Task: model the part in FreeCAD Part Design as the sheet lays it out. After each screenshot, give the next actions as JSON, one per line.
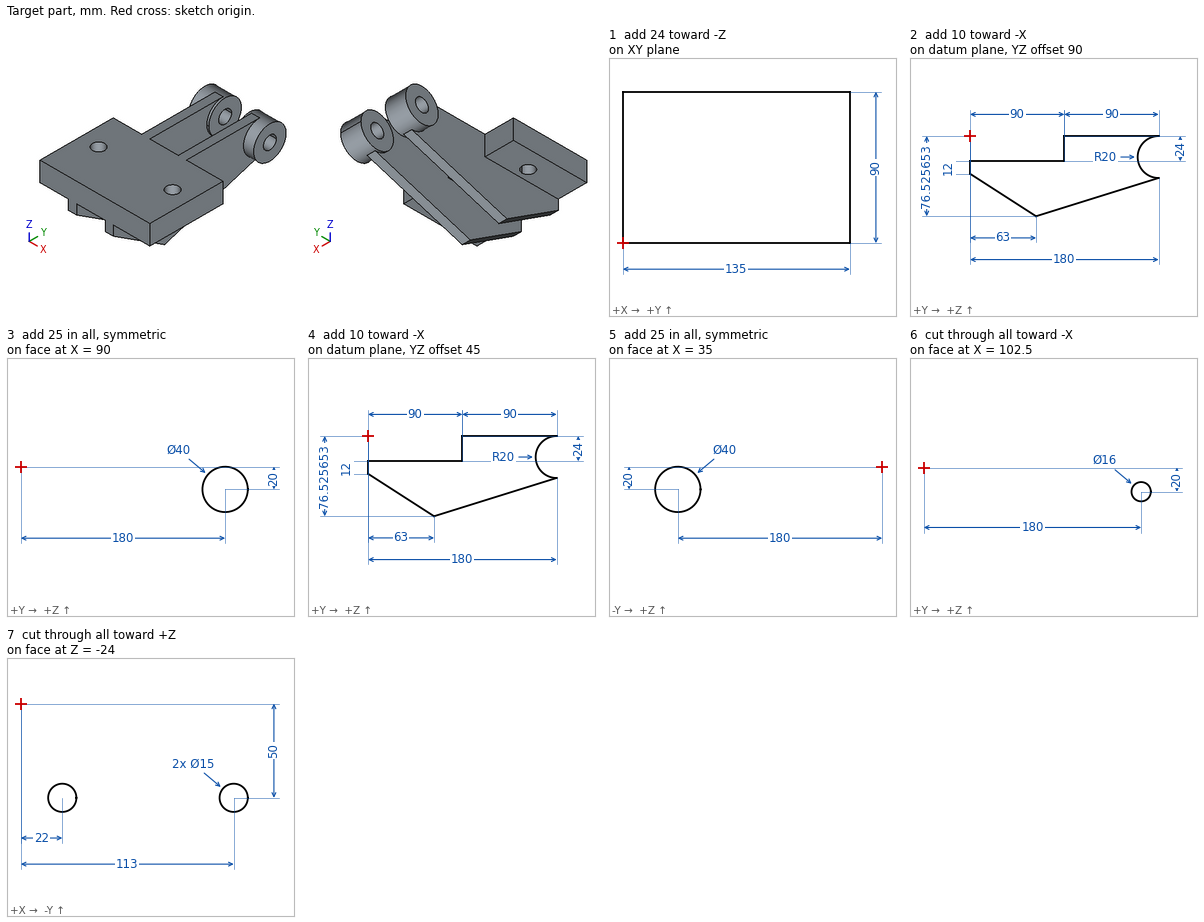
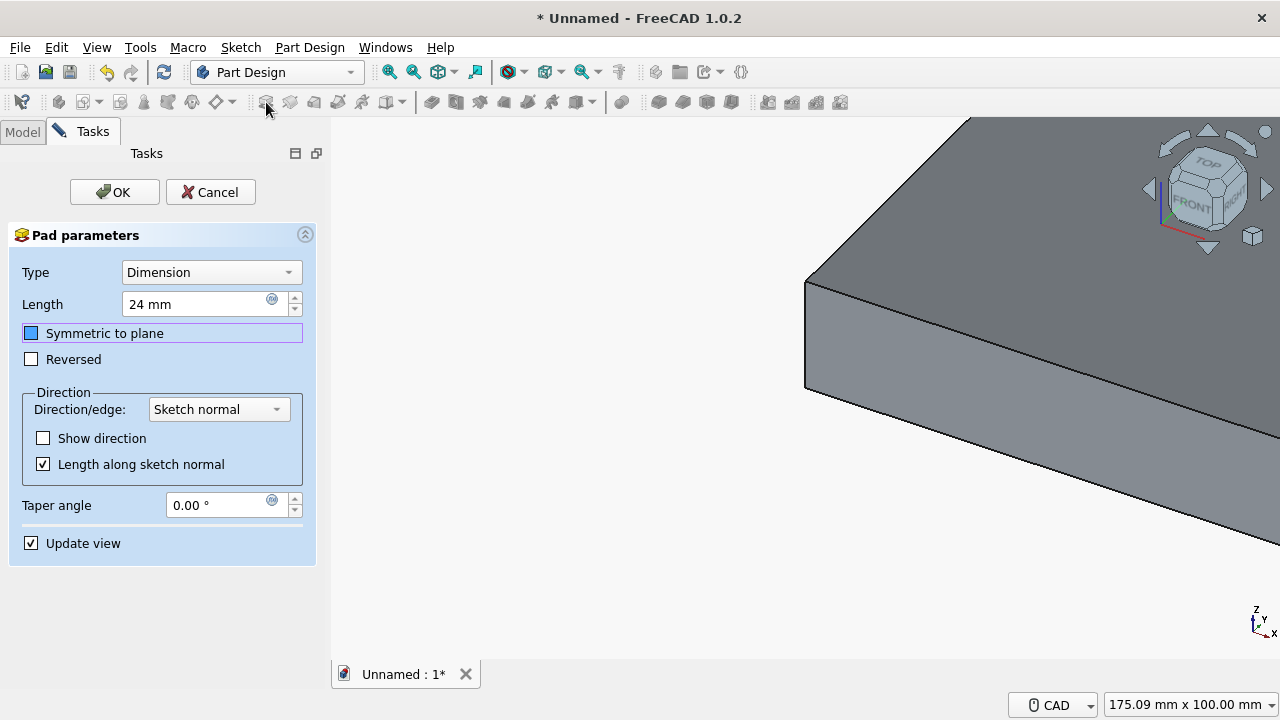
{"action": "left_click", "coordinate": [30, 359]}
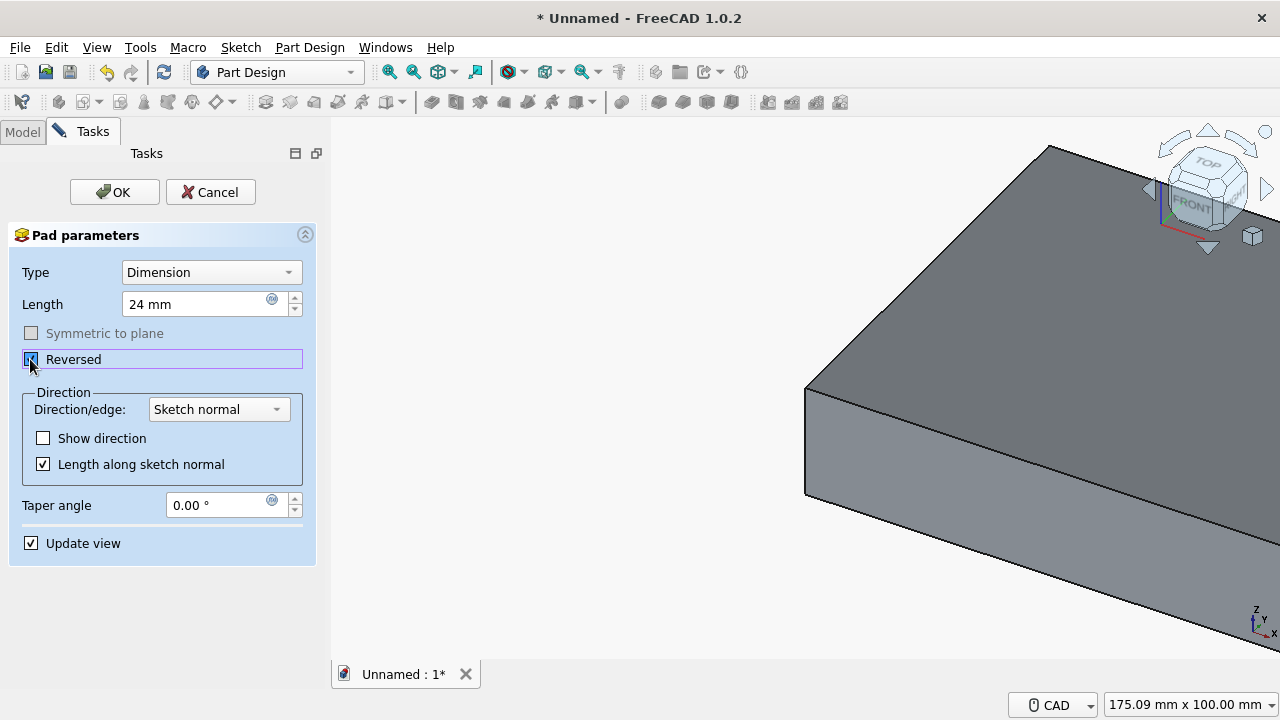
{"action": "left_click", "coordinate": [115, 192]}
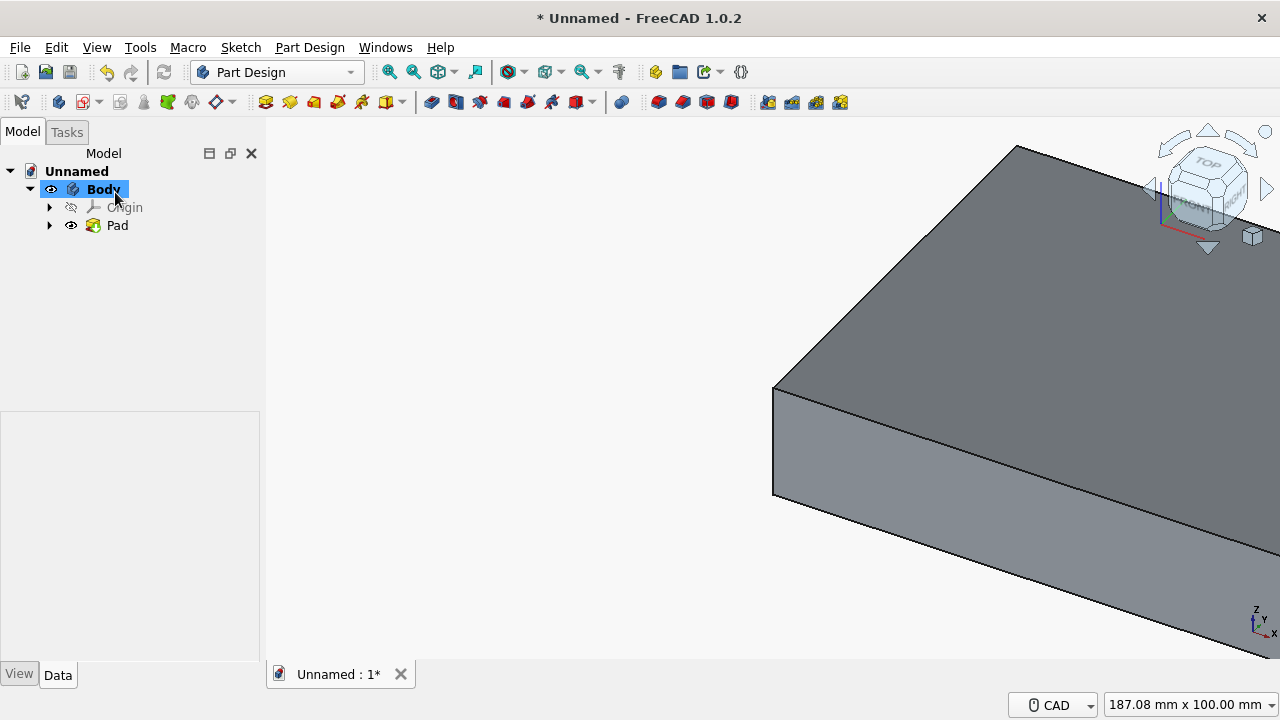
{"action": "left_click", "coordinate": [390, 72]}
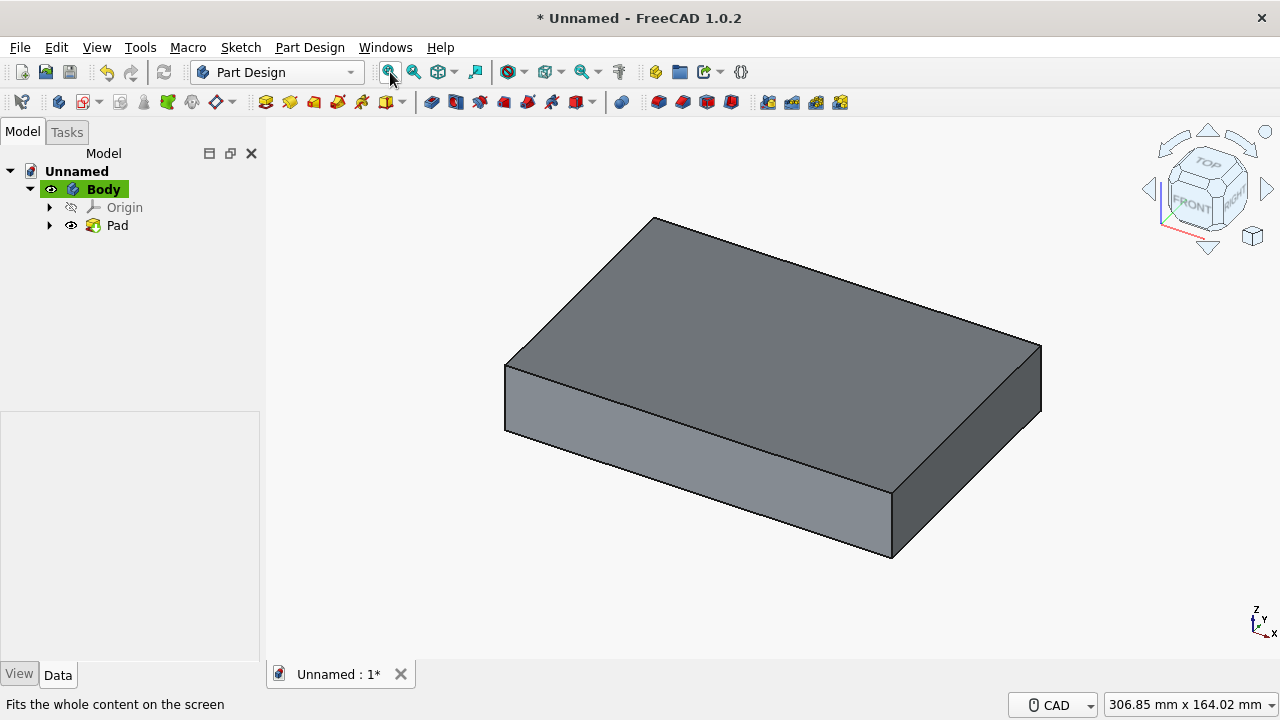
{"action": "left_click", "coordinate": [50, 207]}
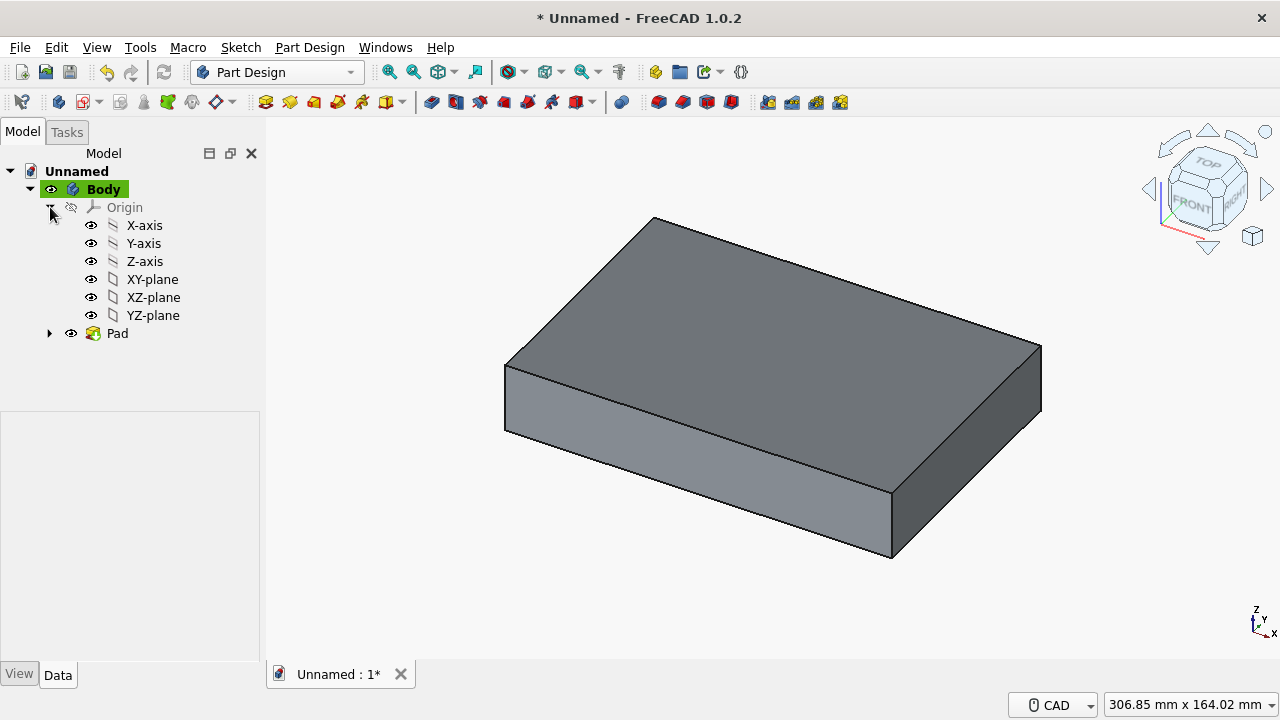
{"action": "left_click", "coordinate": [136, 315]}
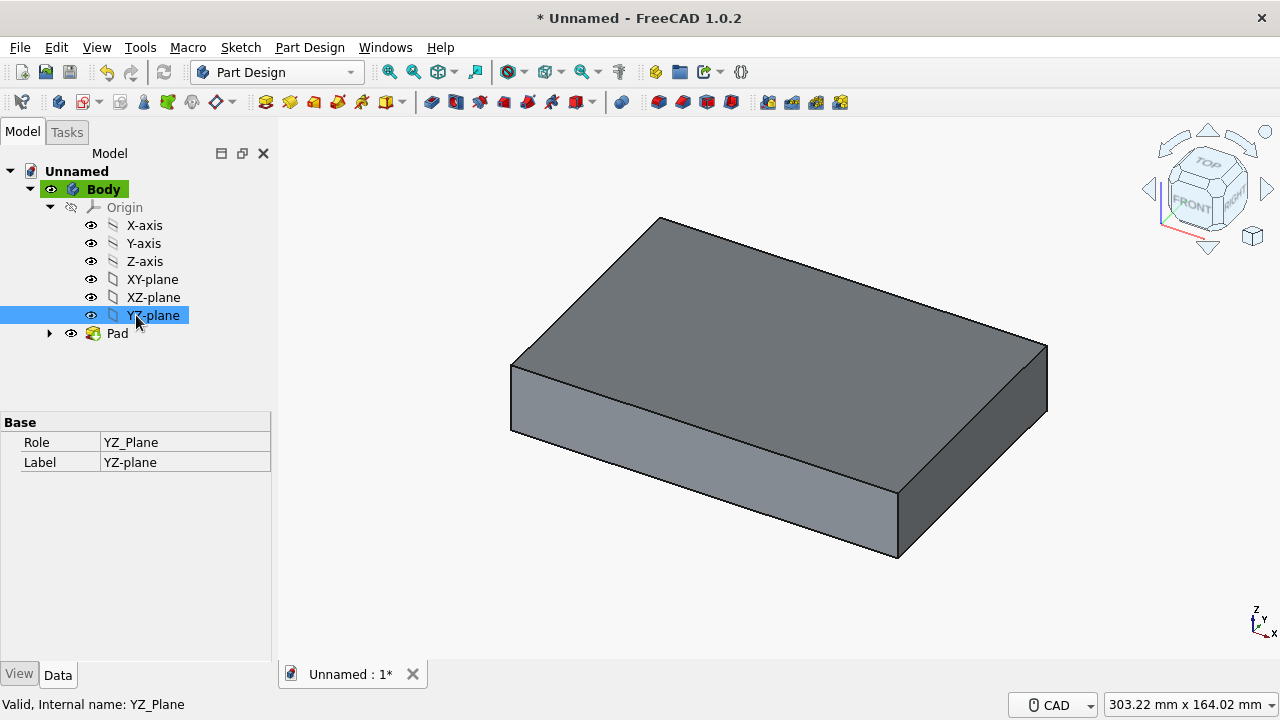
{"action": "left_click", "coordinate": [216, 102]}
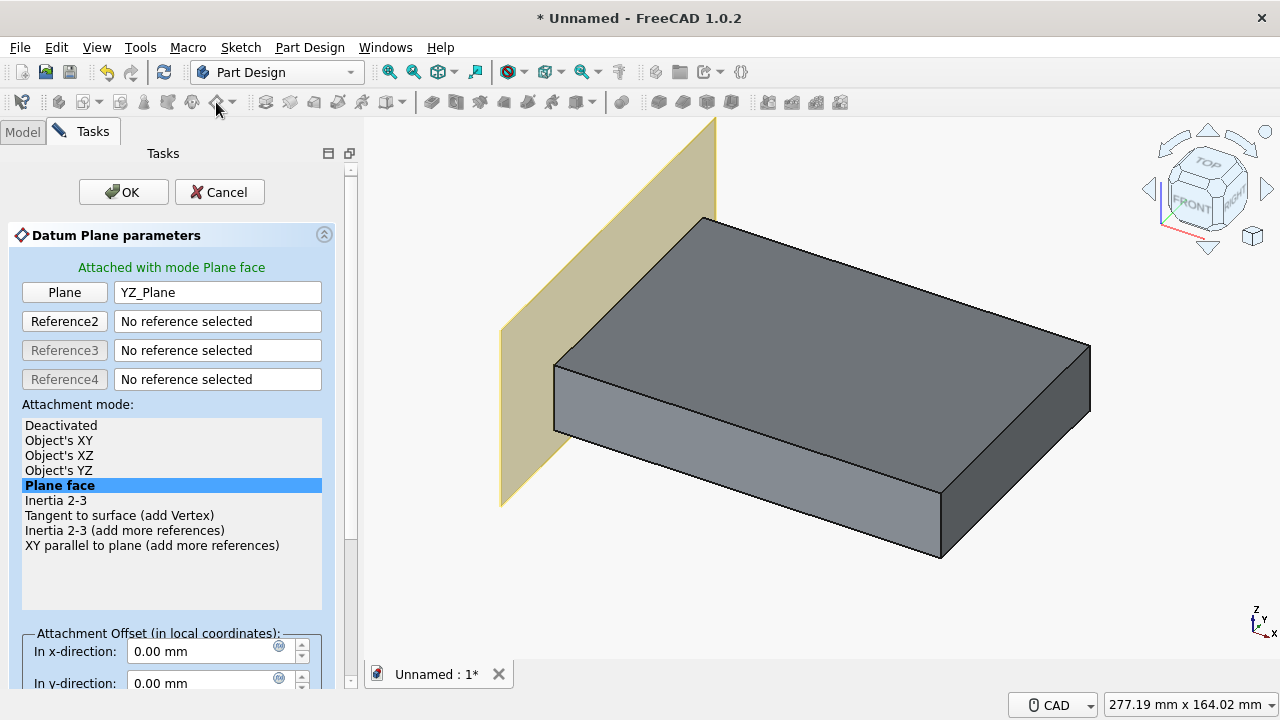
{"action": "scroll", "coordinate": [351, 426], "scroll_direction": "down", "scroll_amount": 2}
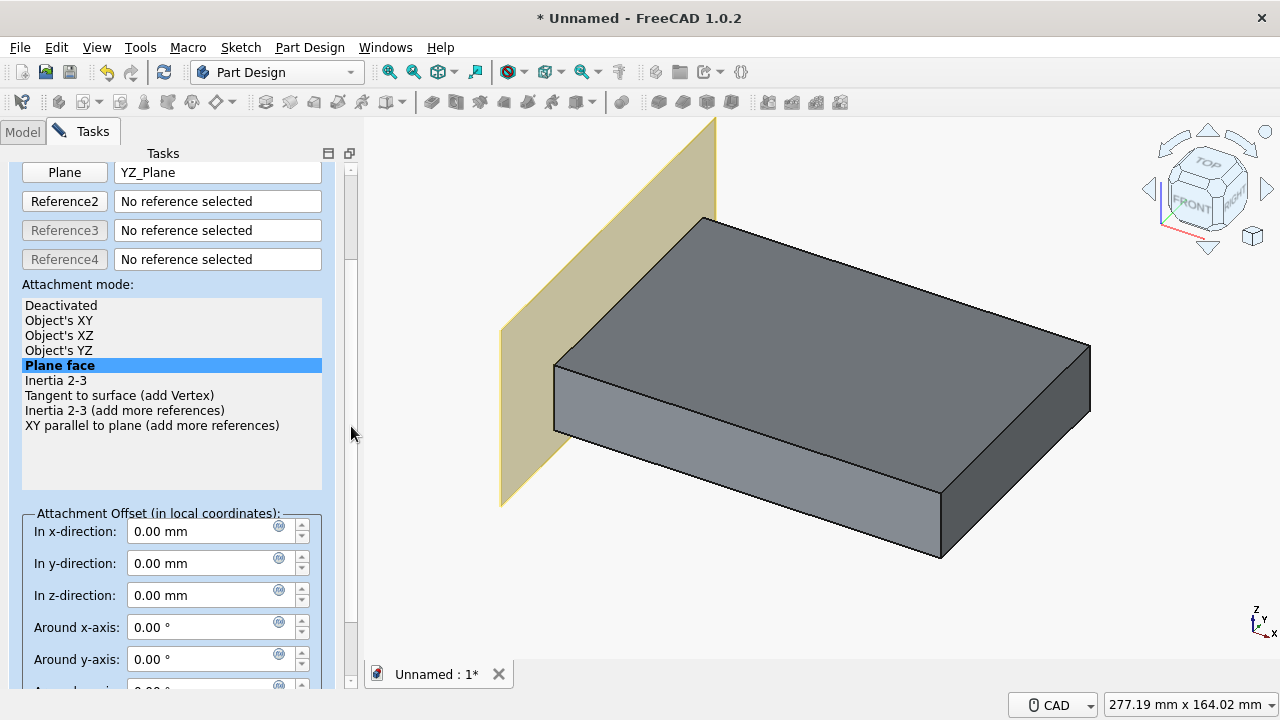
{"action": "triple_click", "coordinate": [210, 595]}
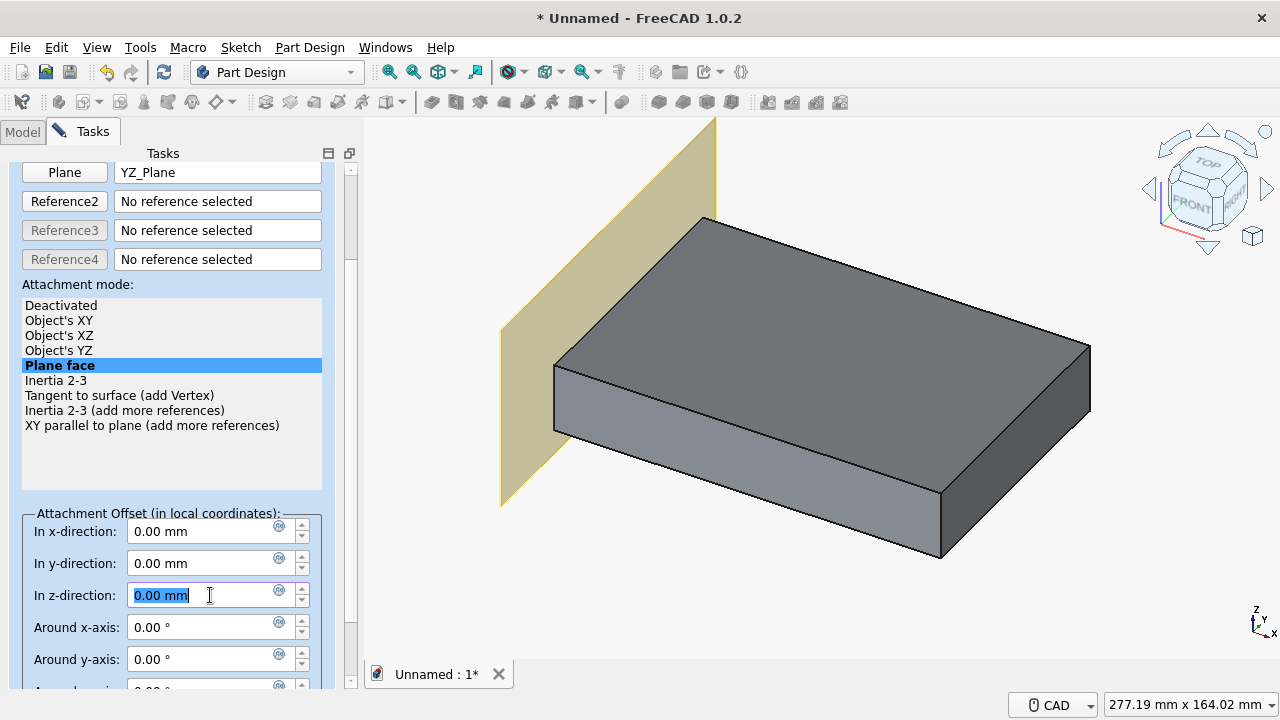
{"action": "type", "text": "90"}
{"action": "key", "text": "Tab"}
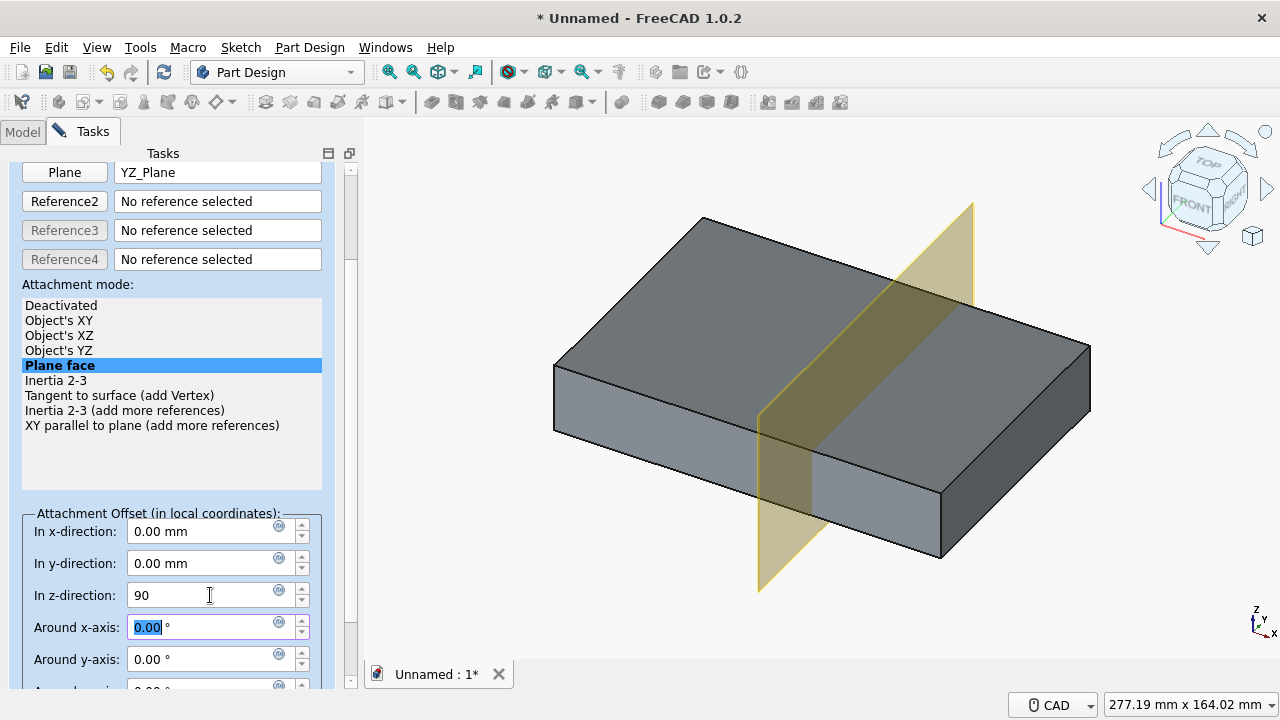
{"action": "scroll", "coordinate": [351, 426], "scroll_direction": "up", "scroll_amount": 3}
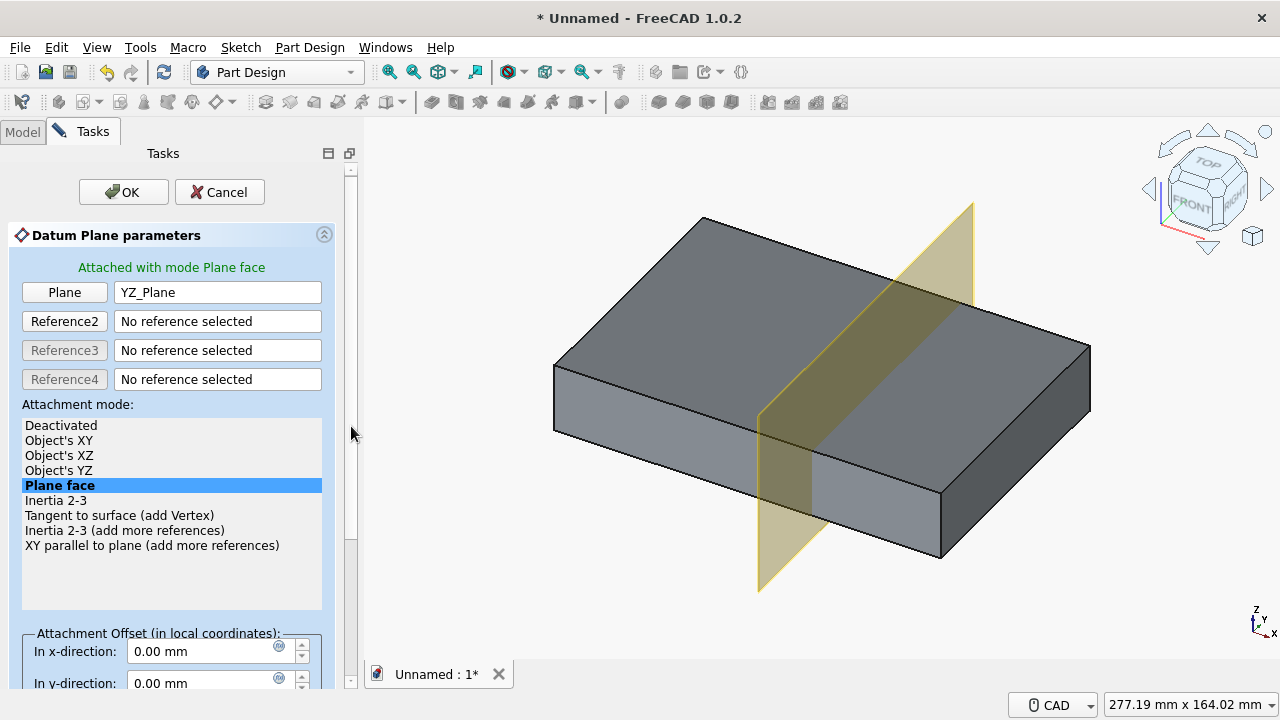
{"action": "left_click", "coordinate": [124, 192]}